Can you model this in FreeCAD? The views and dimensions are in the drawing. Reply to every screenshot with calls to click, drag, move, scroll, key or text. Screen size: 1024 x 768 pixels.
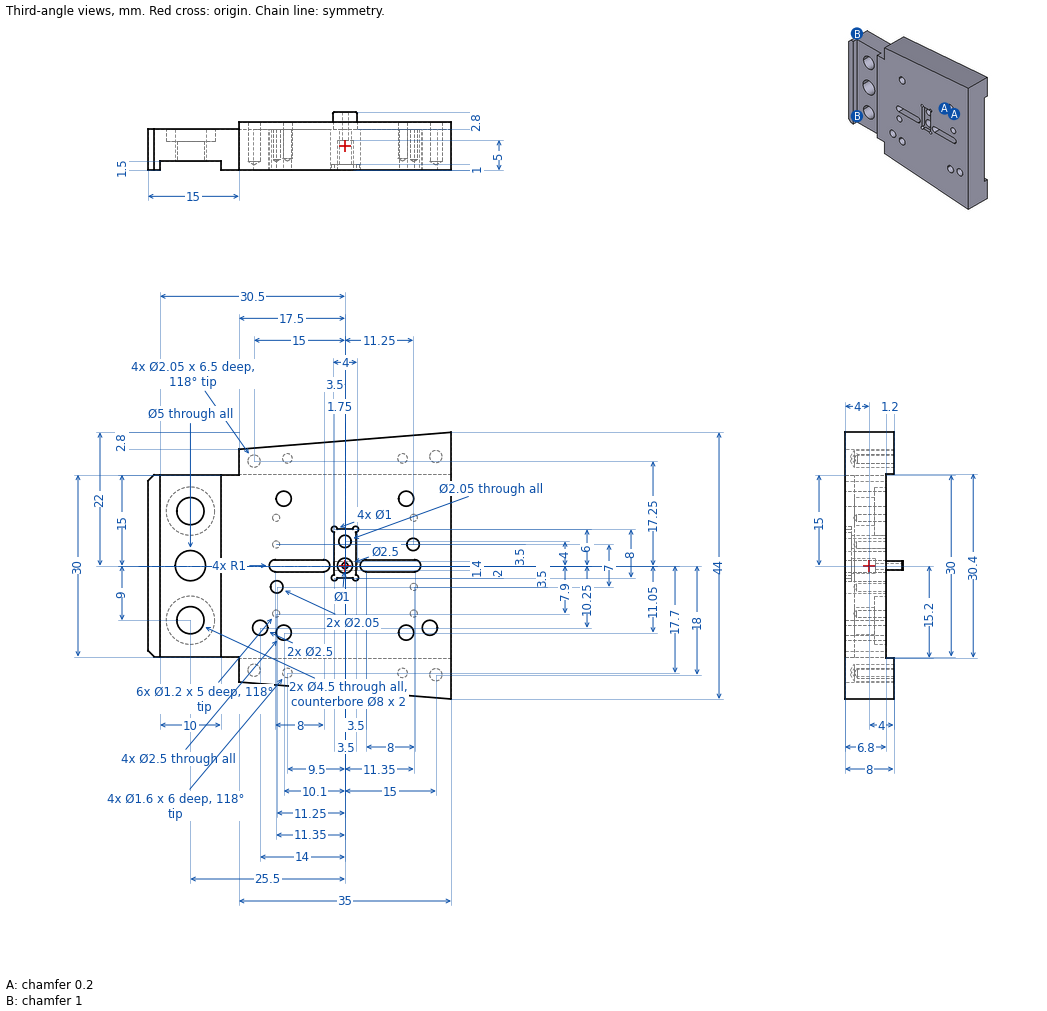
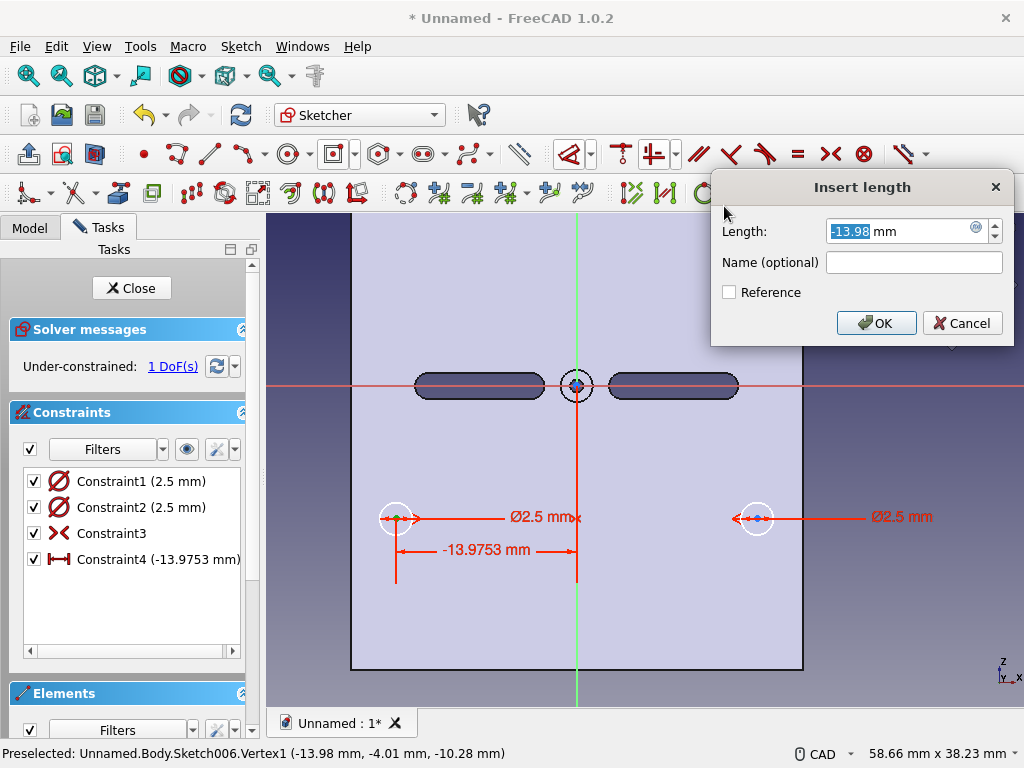
text(-14)
key(Return)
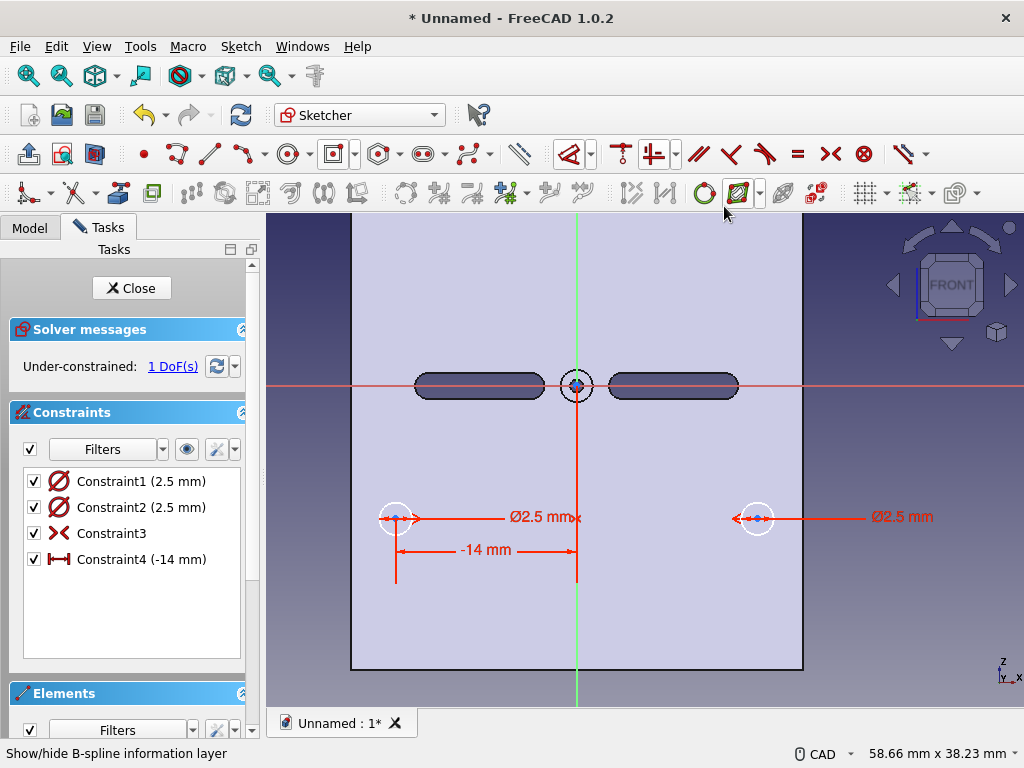
click(396, 519)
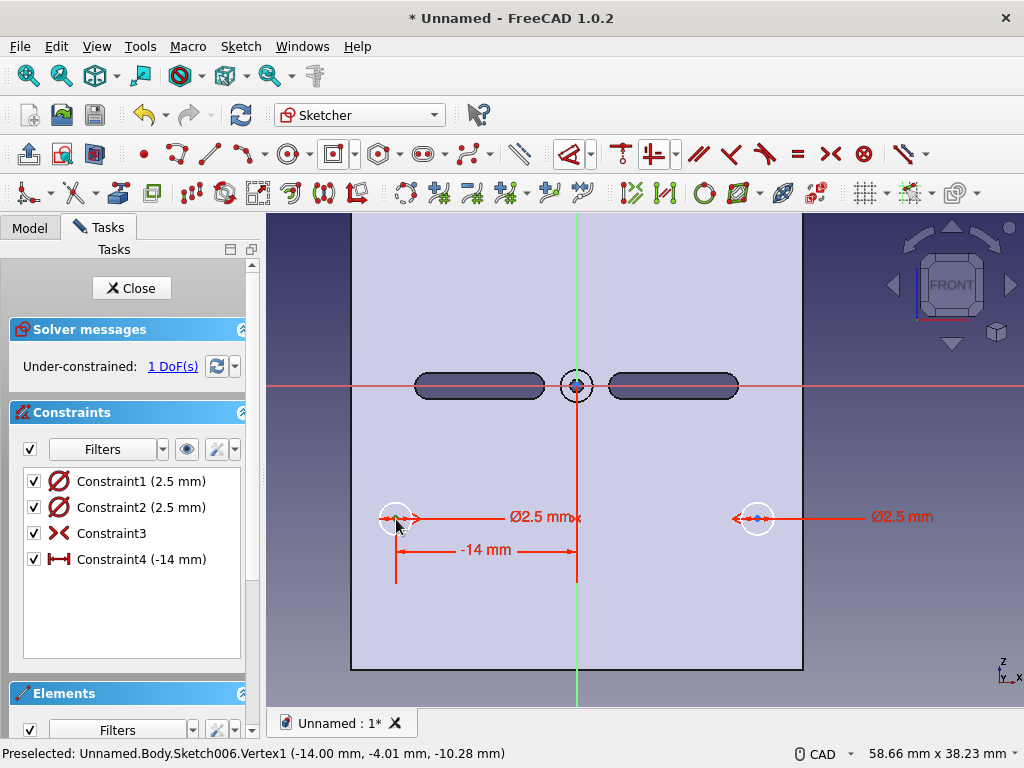
click(590, 154)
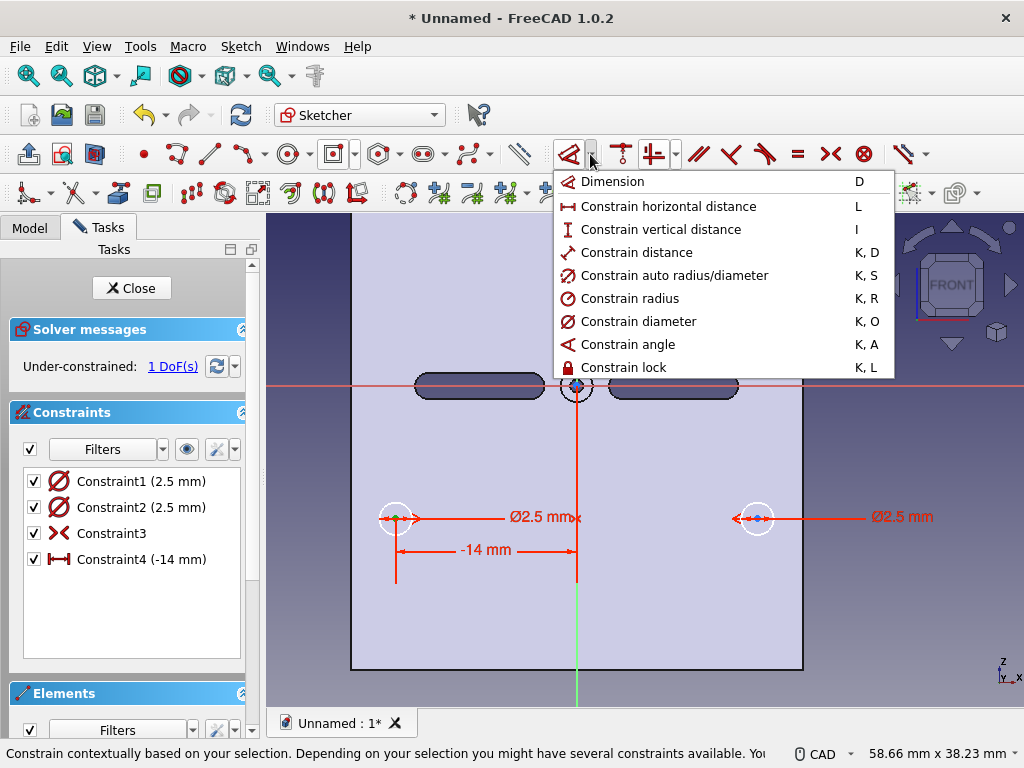
click(724, 230)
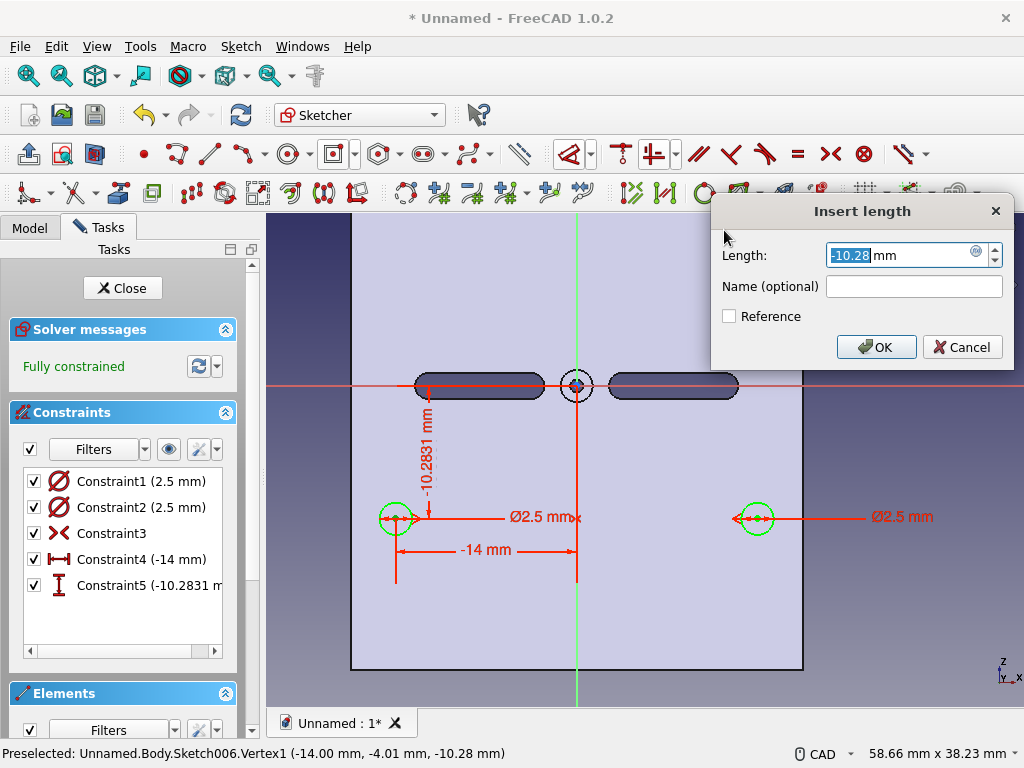
text(-10.25)
key(Return)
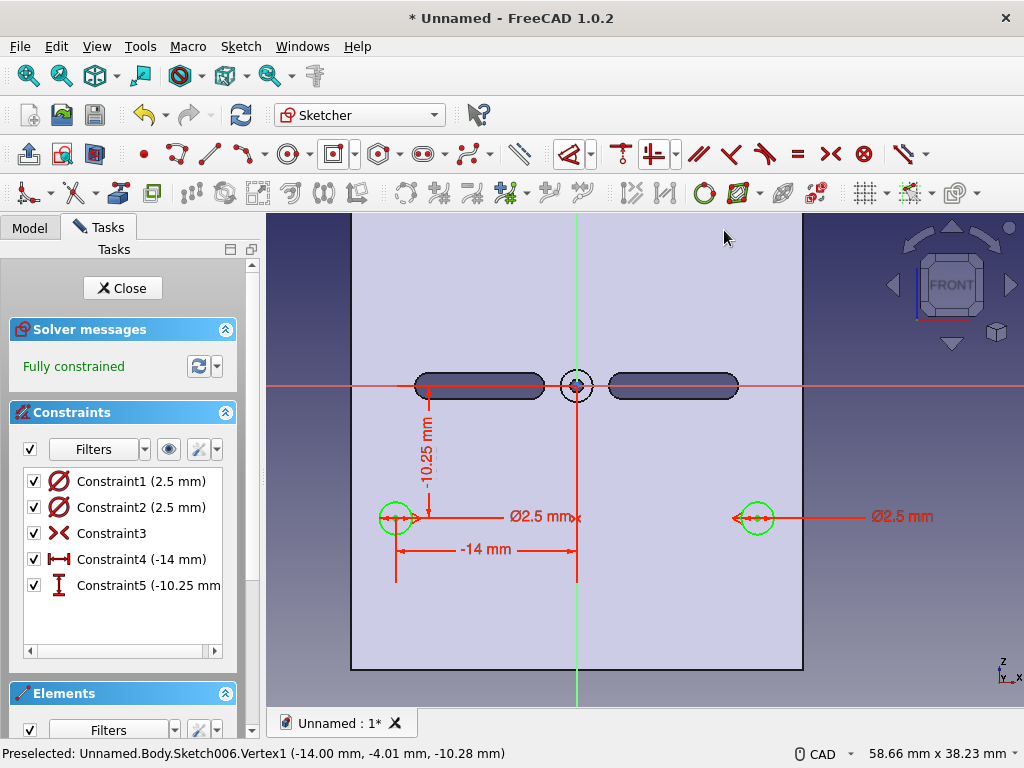
click(123, 288)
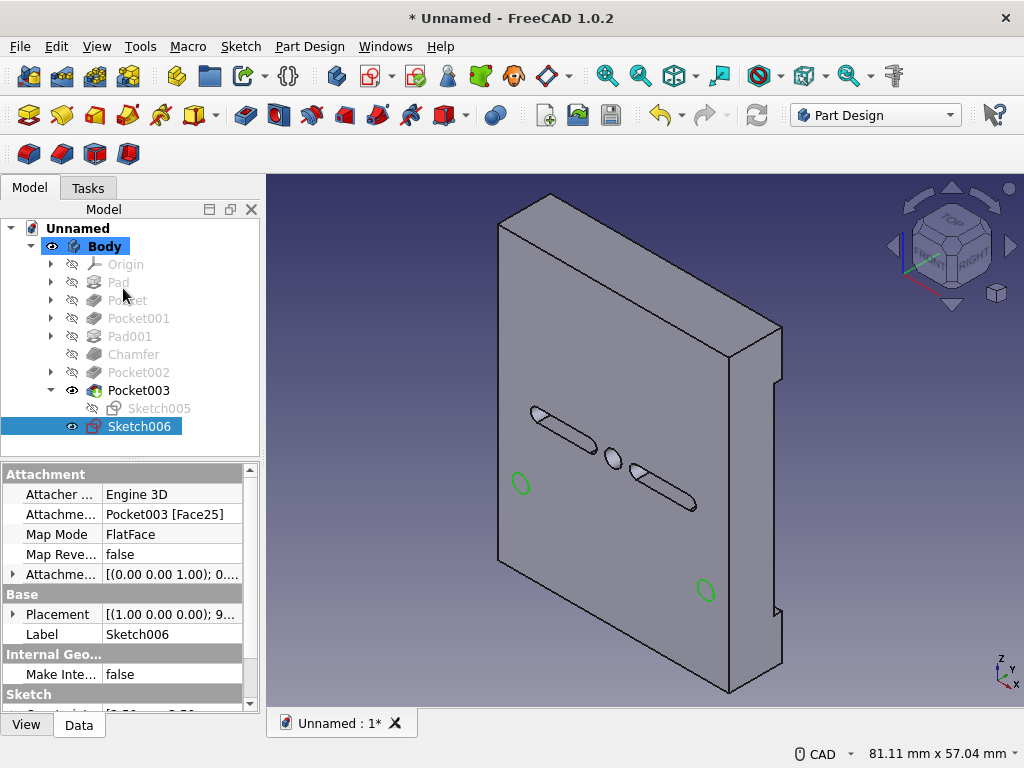
click(246, 116)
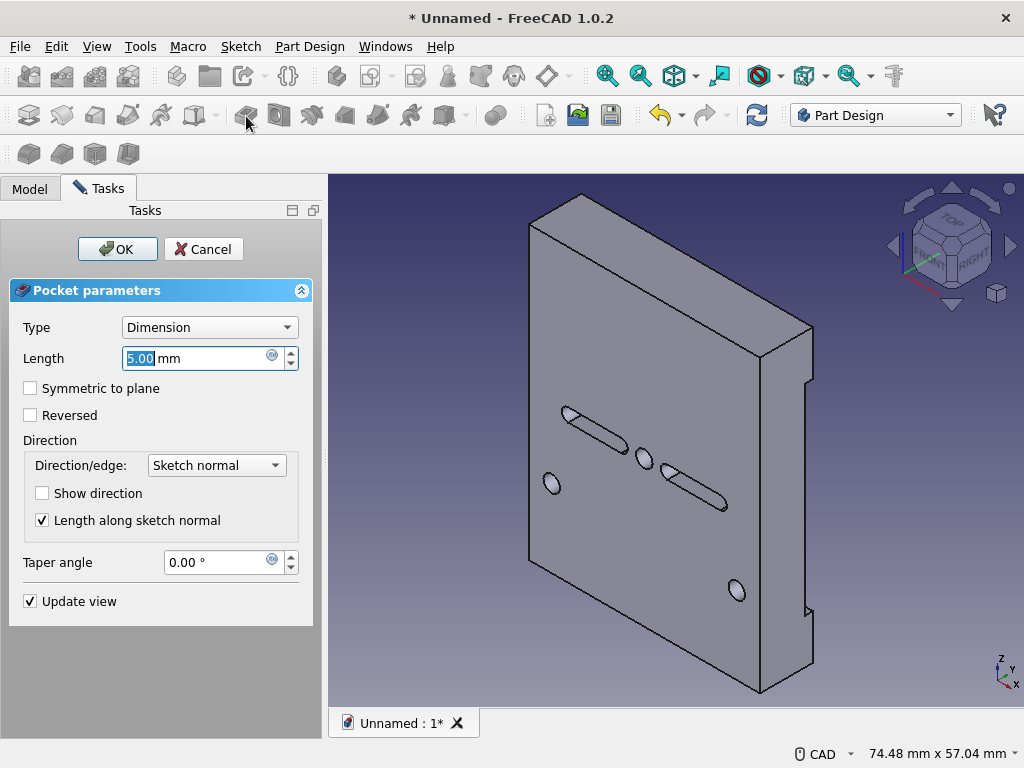
click(210, 328)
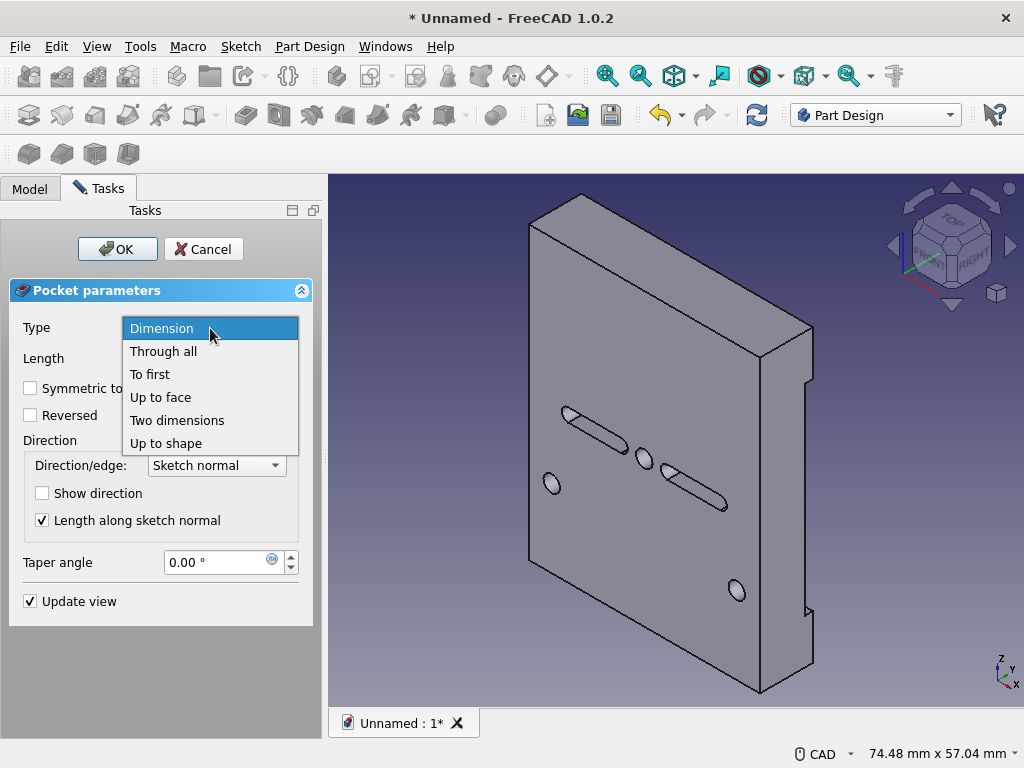
click(208, 352)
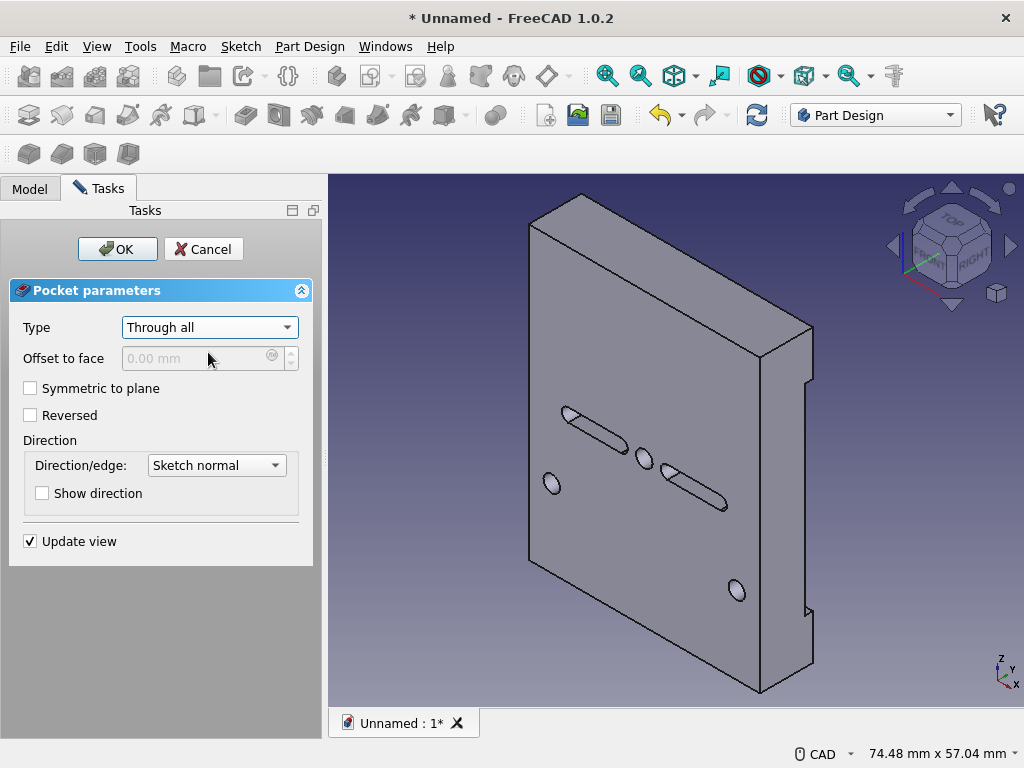
click(118, 249)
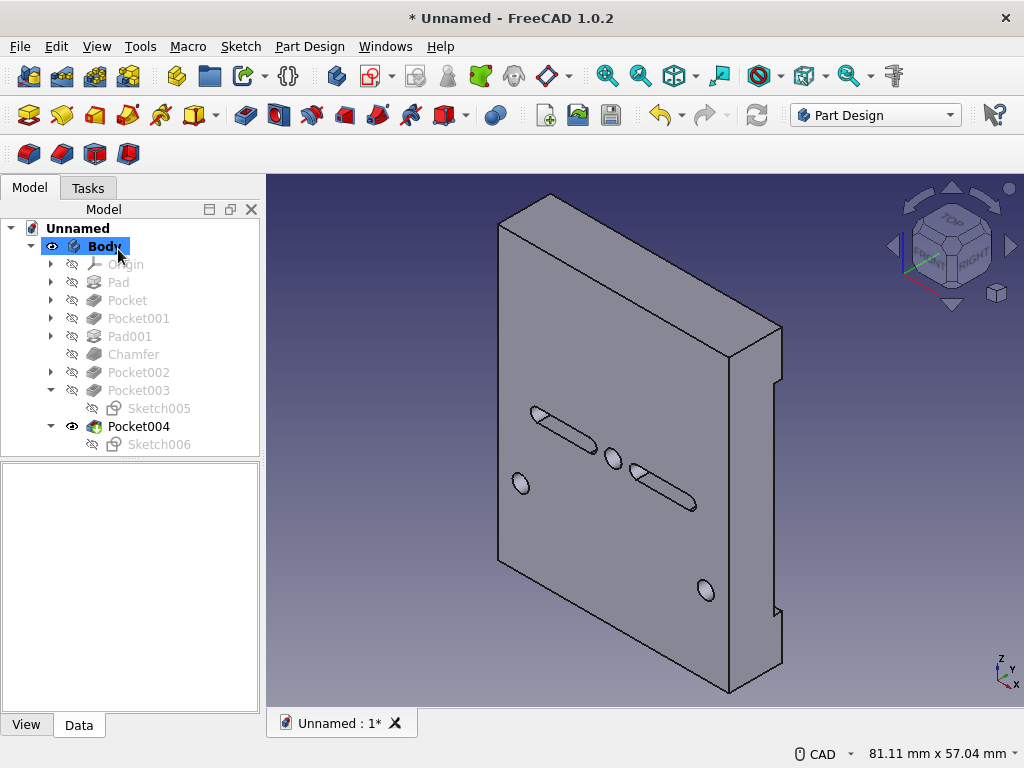
click(613, 554)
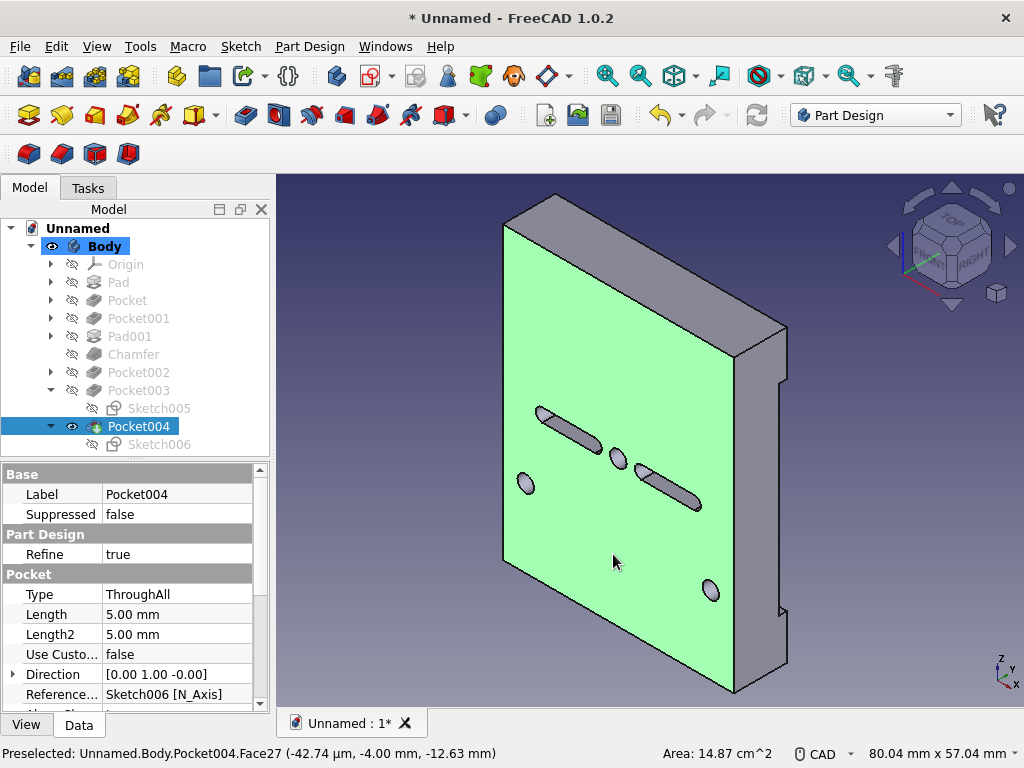
click(370, 76)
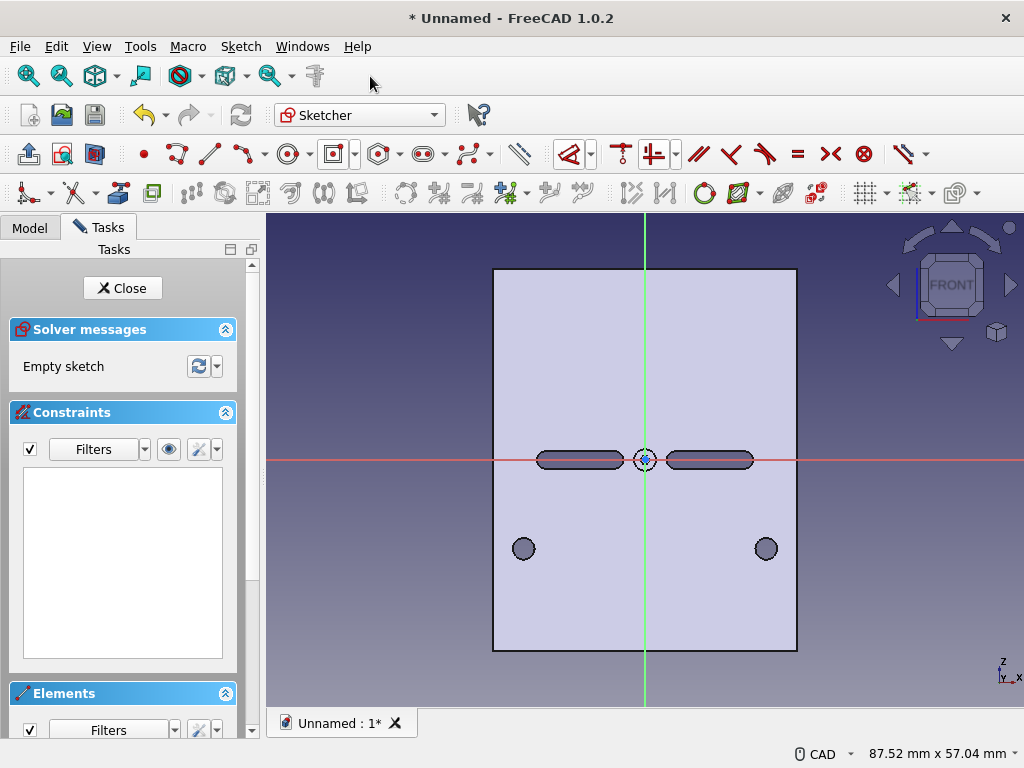
scroll(667, 437, up, 7)